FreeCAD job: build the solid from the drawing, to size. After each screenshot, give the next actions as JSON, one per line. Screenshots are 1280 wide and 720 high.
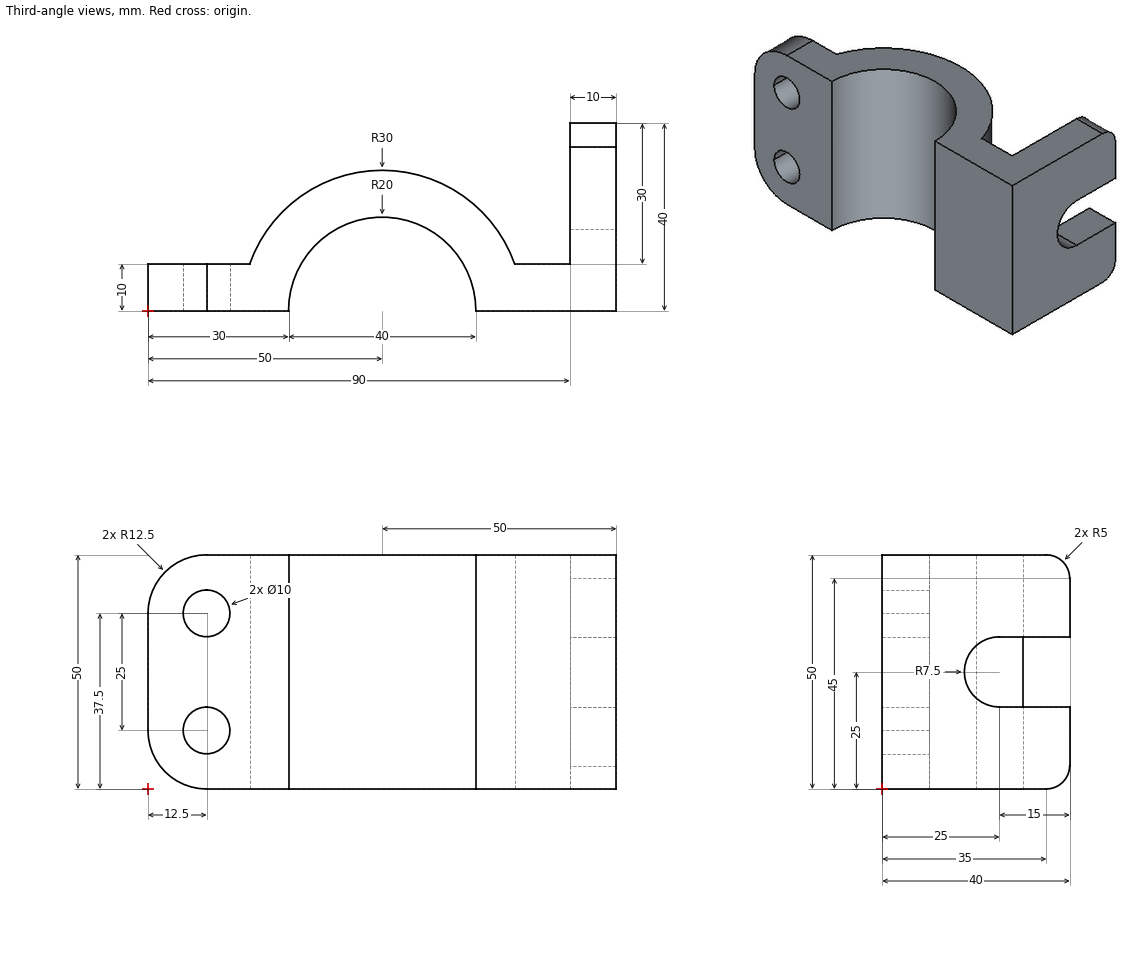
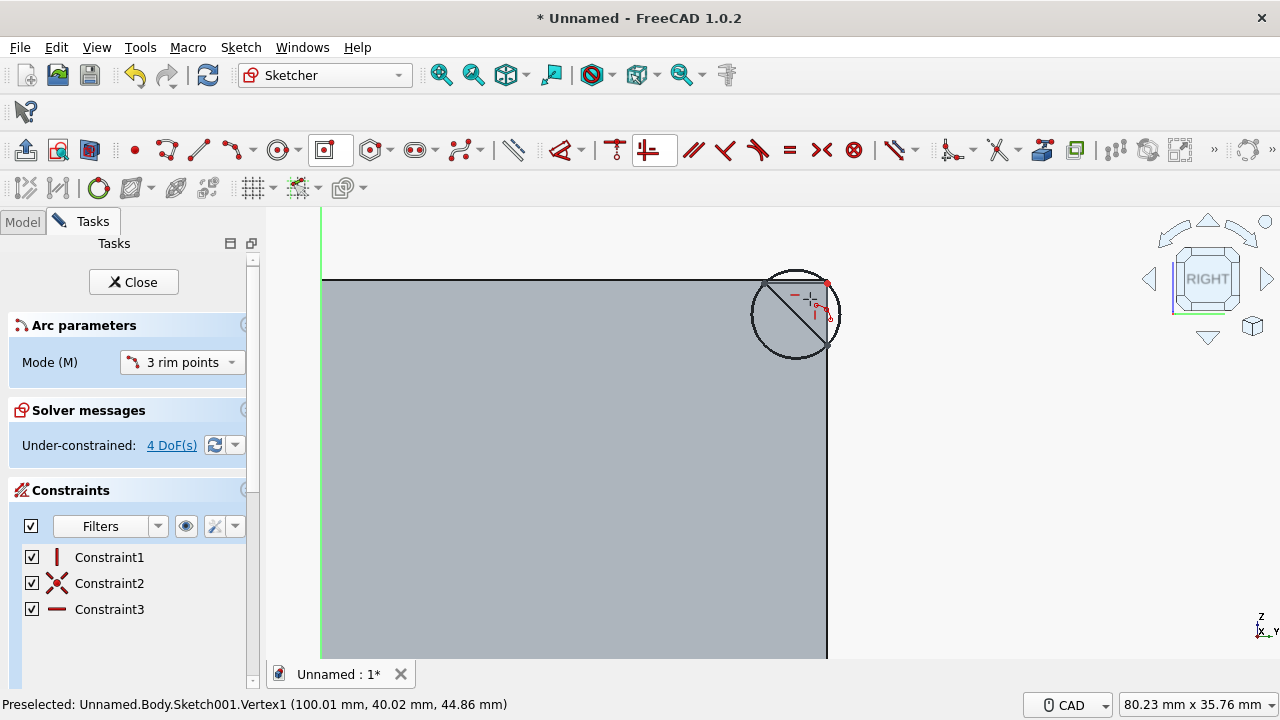
{"action": "left_click", "coordinate": [808, 299]}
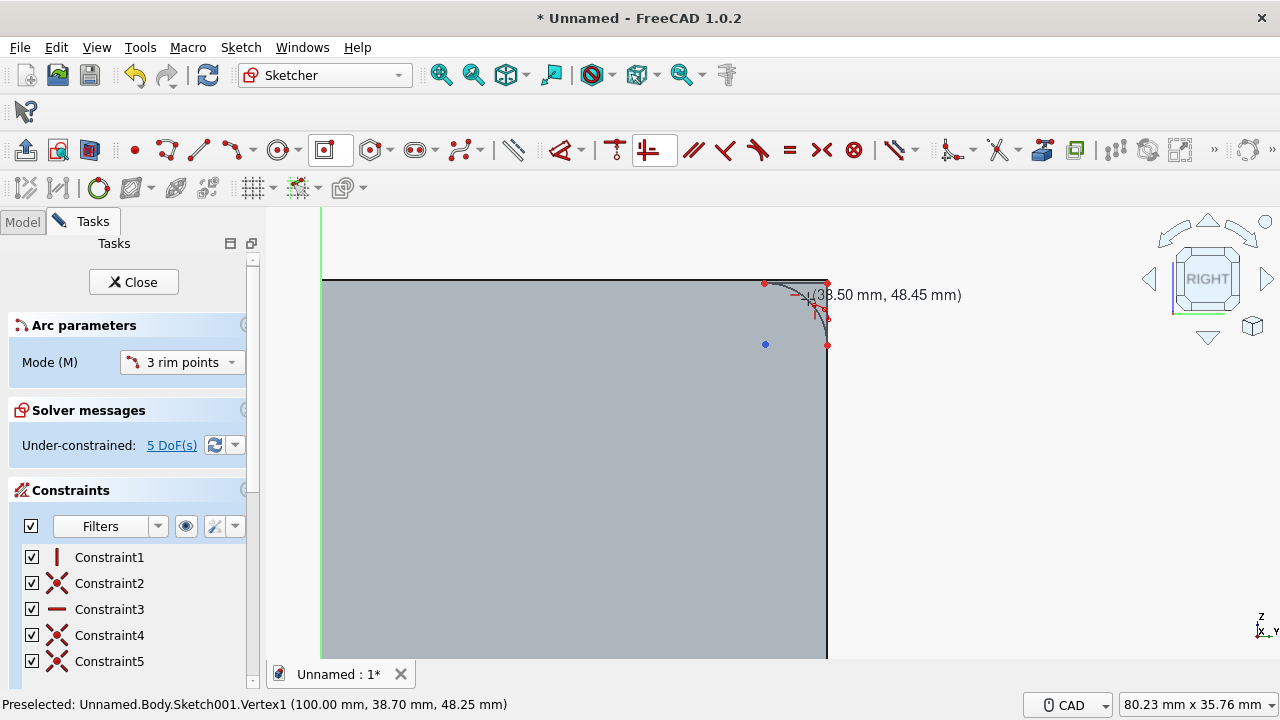
{"action": "left_click", "coordinate": [168, 150]}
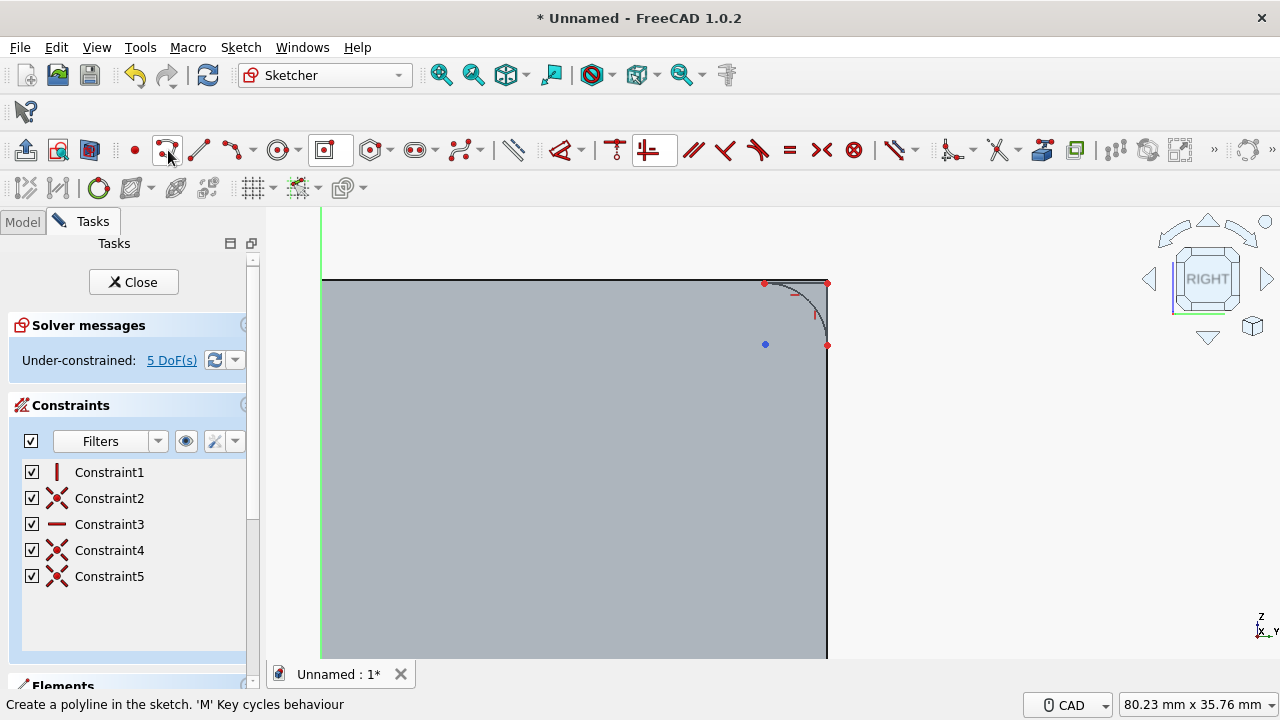
{"action": "scroll", "coordinate": [811, 300], "scroll_direction": "down", "scroll_amount": 4}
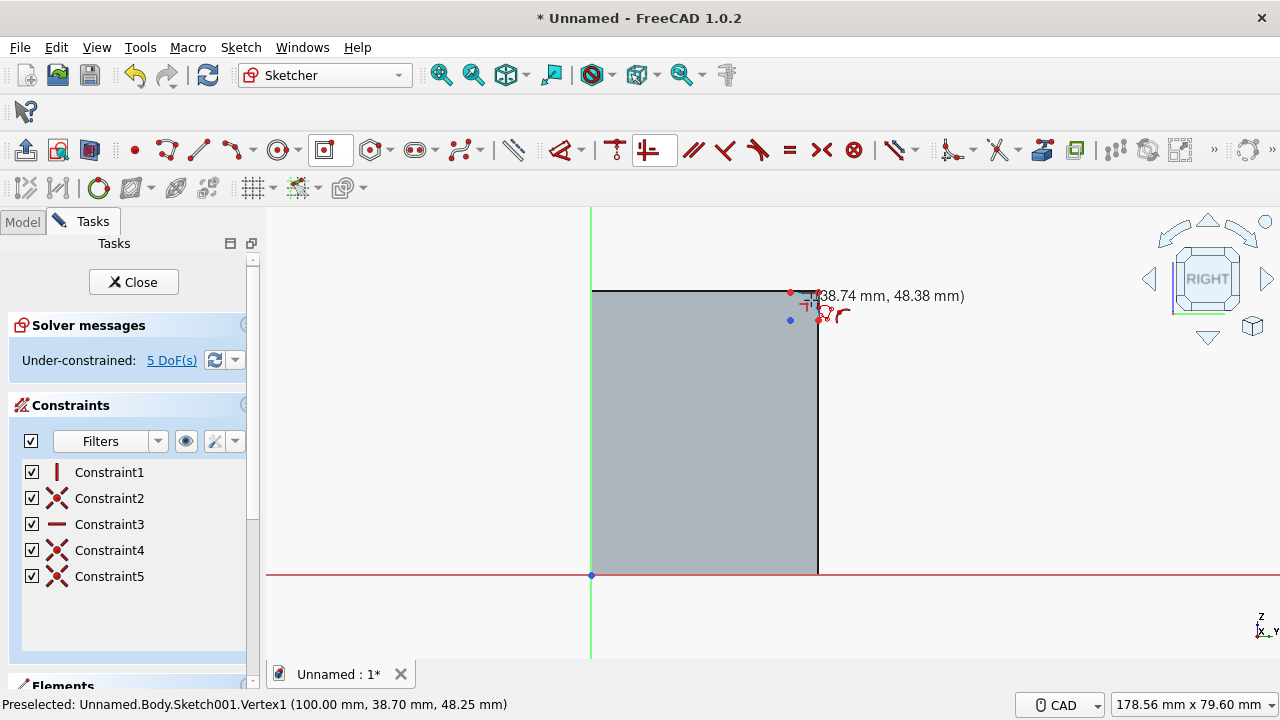
{"action": "left_click", "coordinate": [790, 575]}
{"action": "left_click", "coordinate": [818, 566]}
{"action": "left_click", "coordinate": [818, 547]}
{"action": "right_click", "coordinate": [818, 547]}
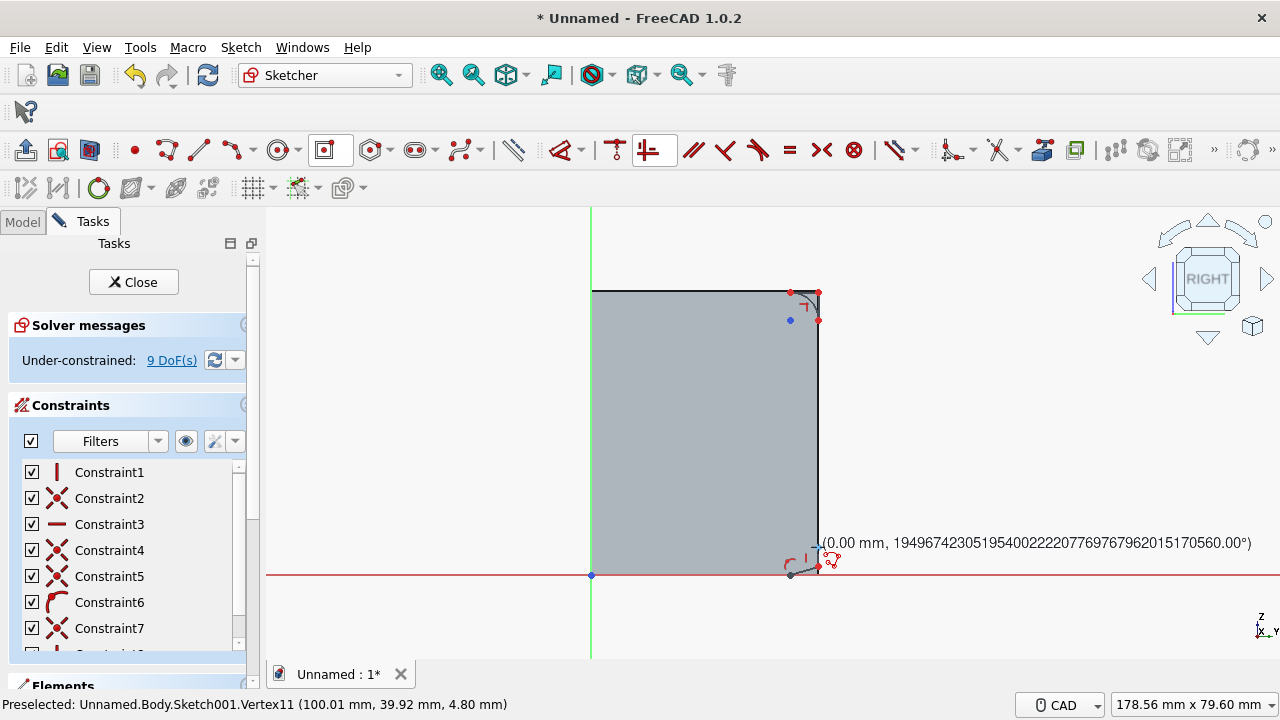
{"action": "left_click", "coordinate": [232, 150]}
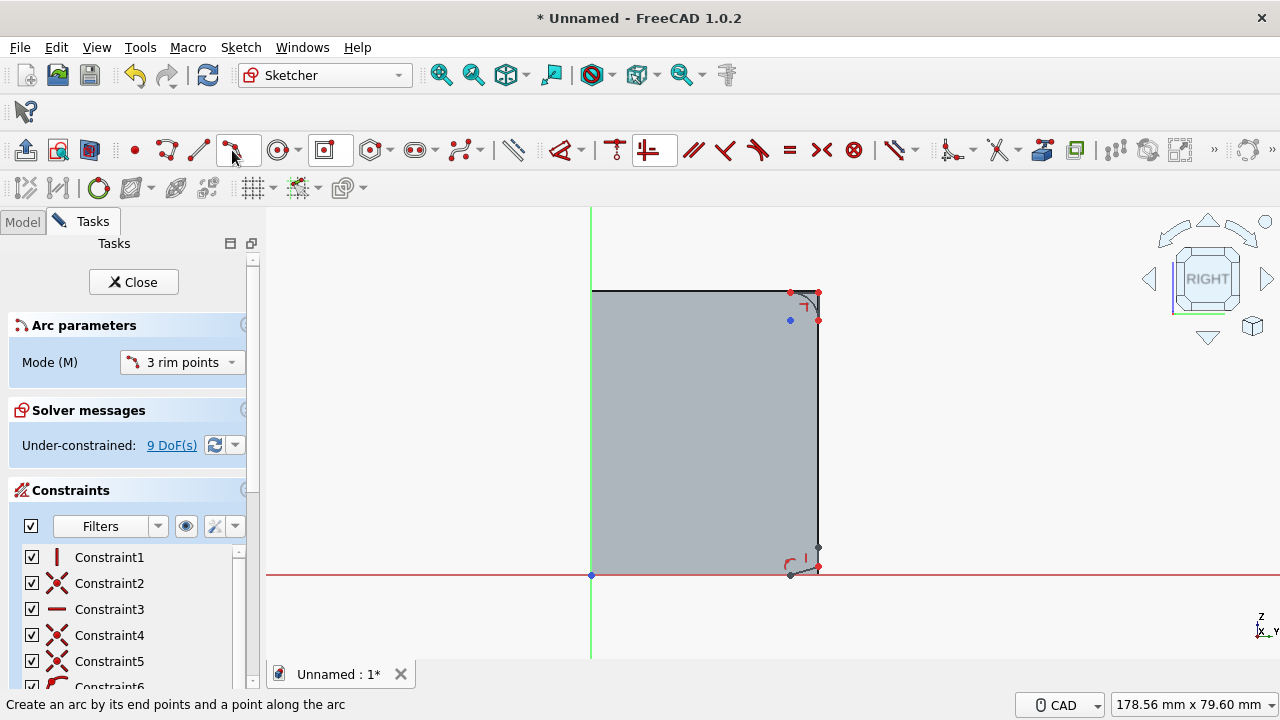
{"action": "left_click", "coordinate": [818, 548]}
{"action": "left_click", "coordinate": [790, 575]}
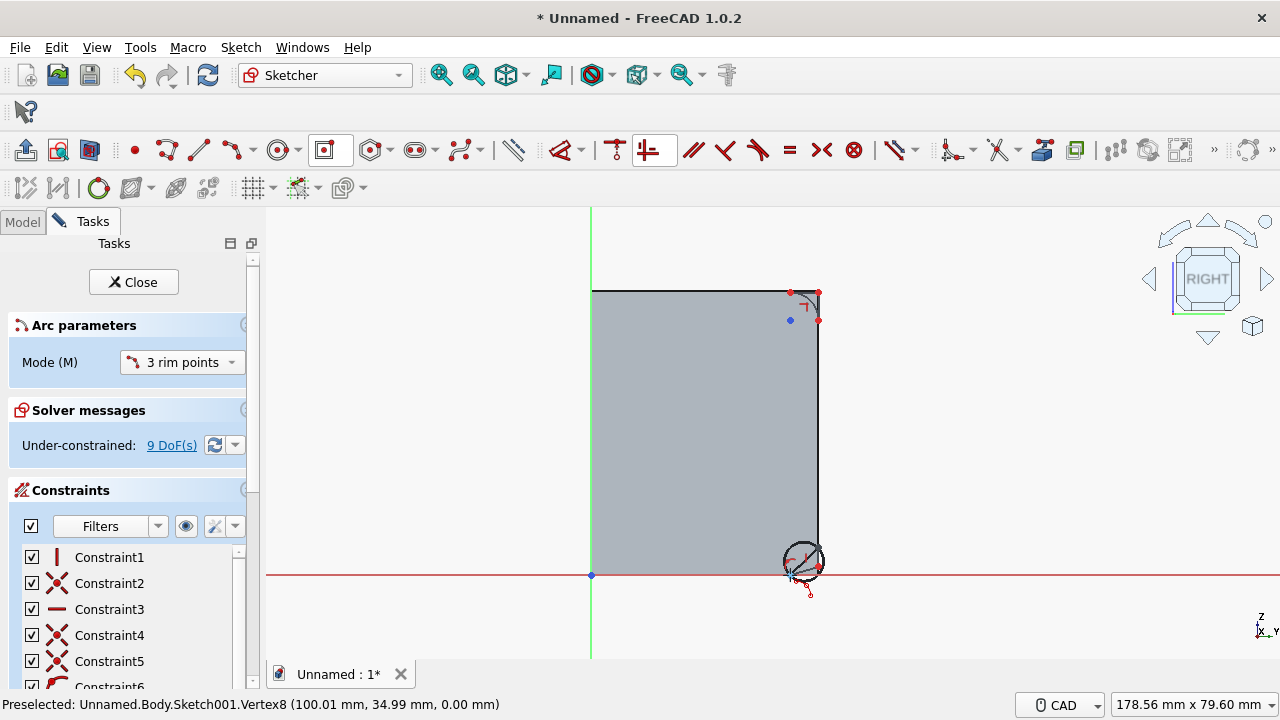
{"action": "scroll", "coordinate": [810, 567], "scroll_direction": "up", "scroll_amount": 4}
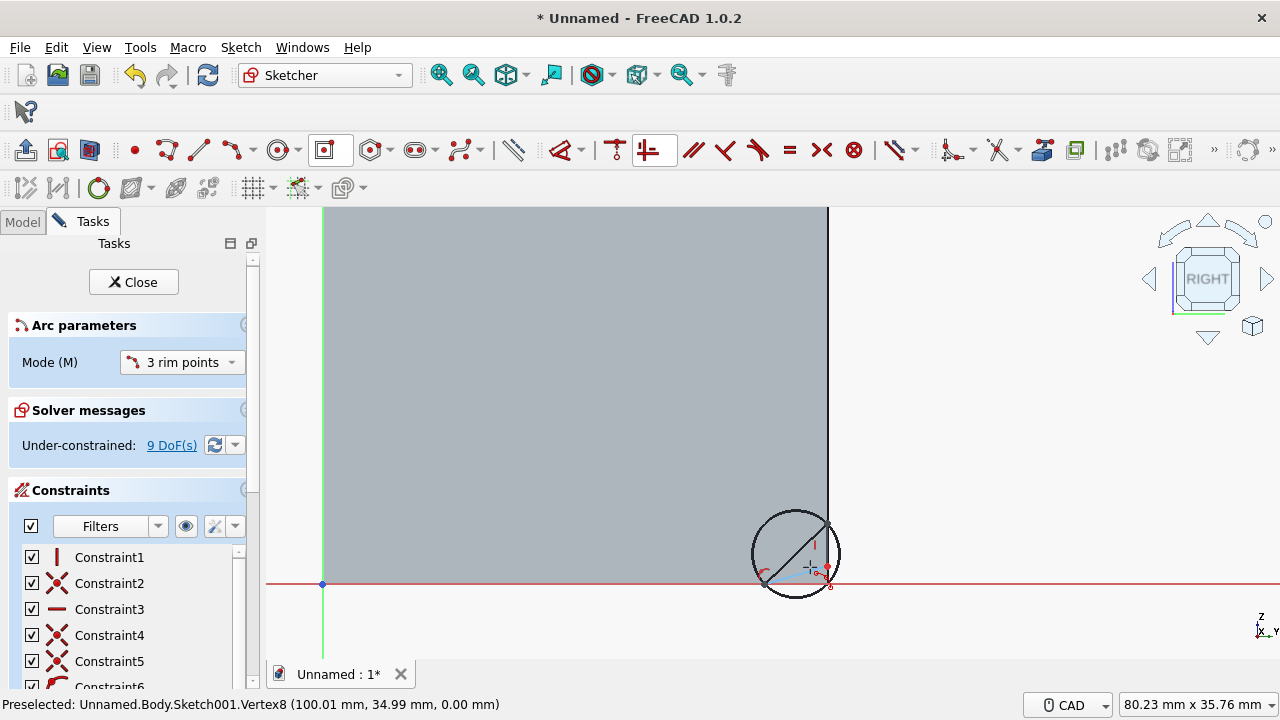
{"action": "left_click", "coordinate": [810, 566]}
{"action": "key", "text": "Escape"}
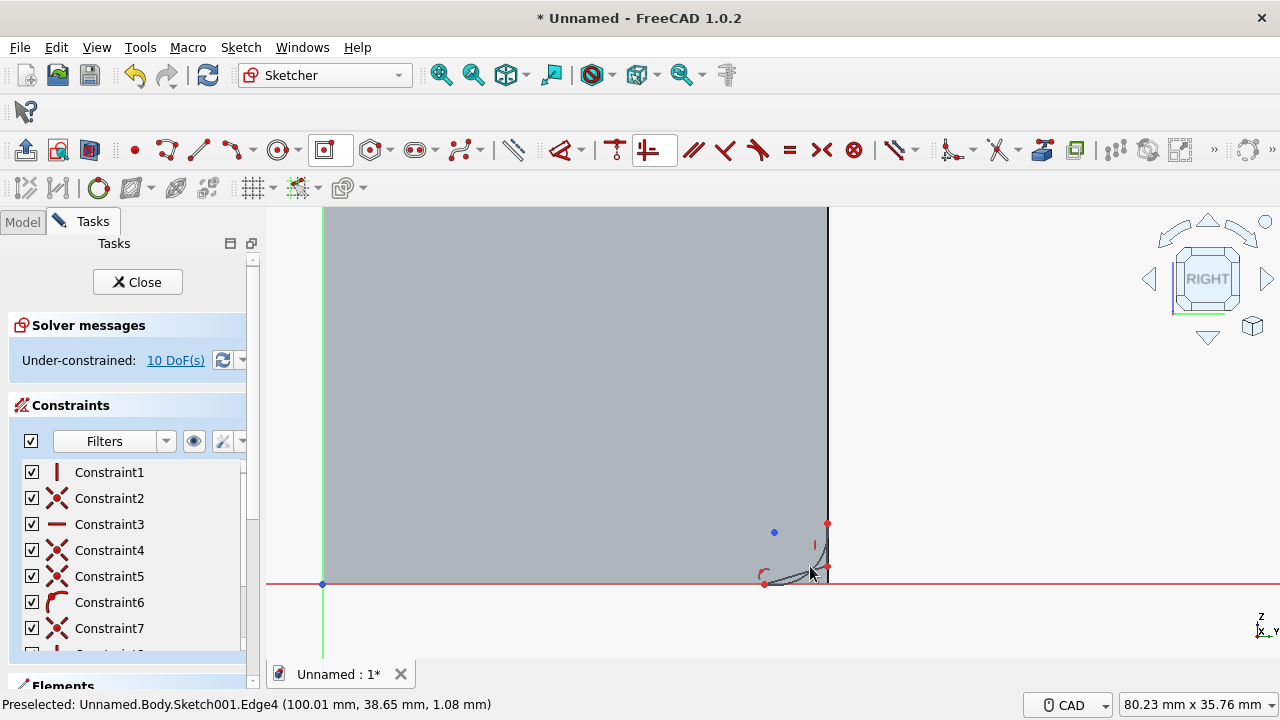
{"action": "scroll", "coordinate": [810, 567], "scroll_direction": "down", "scroll_amount": 4}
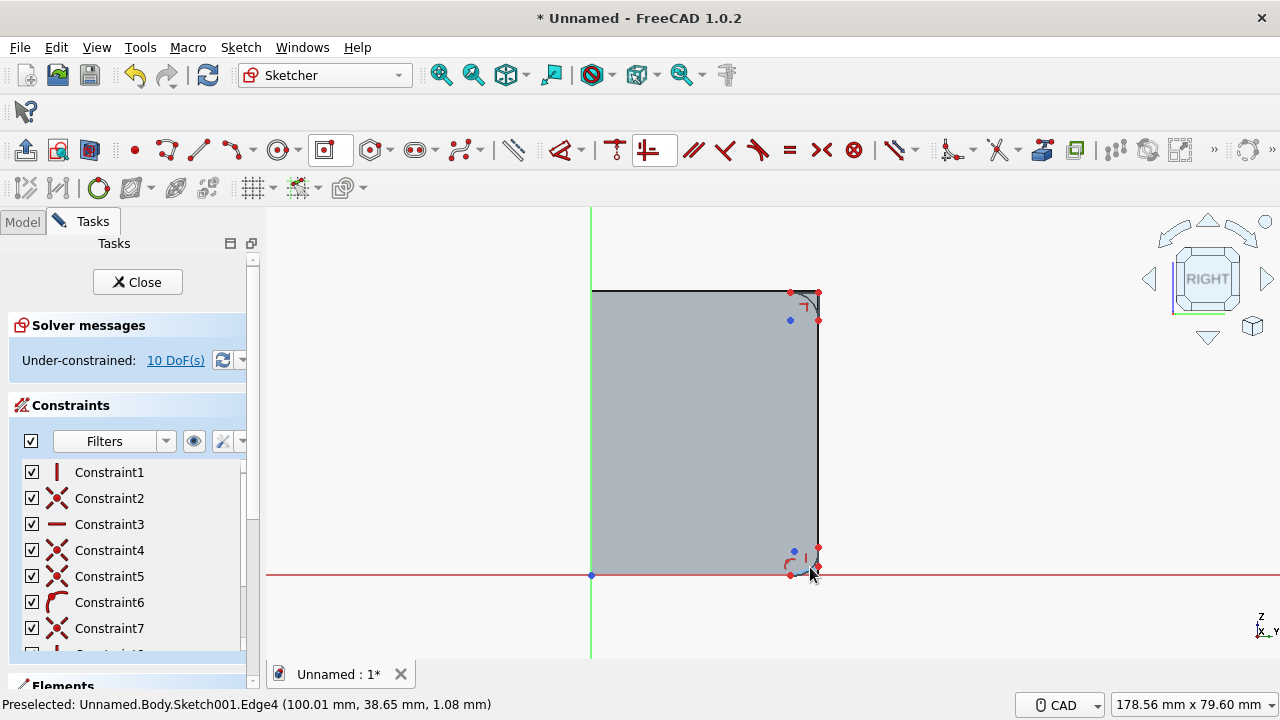
{"action": "scroll", "coordinate": [819, 301], "scroll_direction": "up", "scroll_amount": 5}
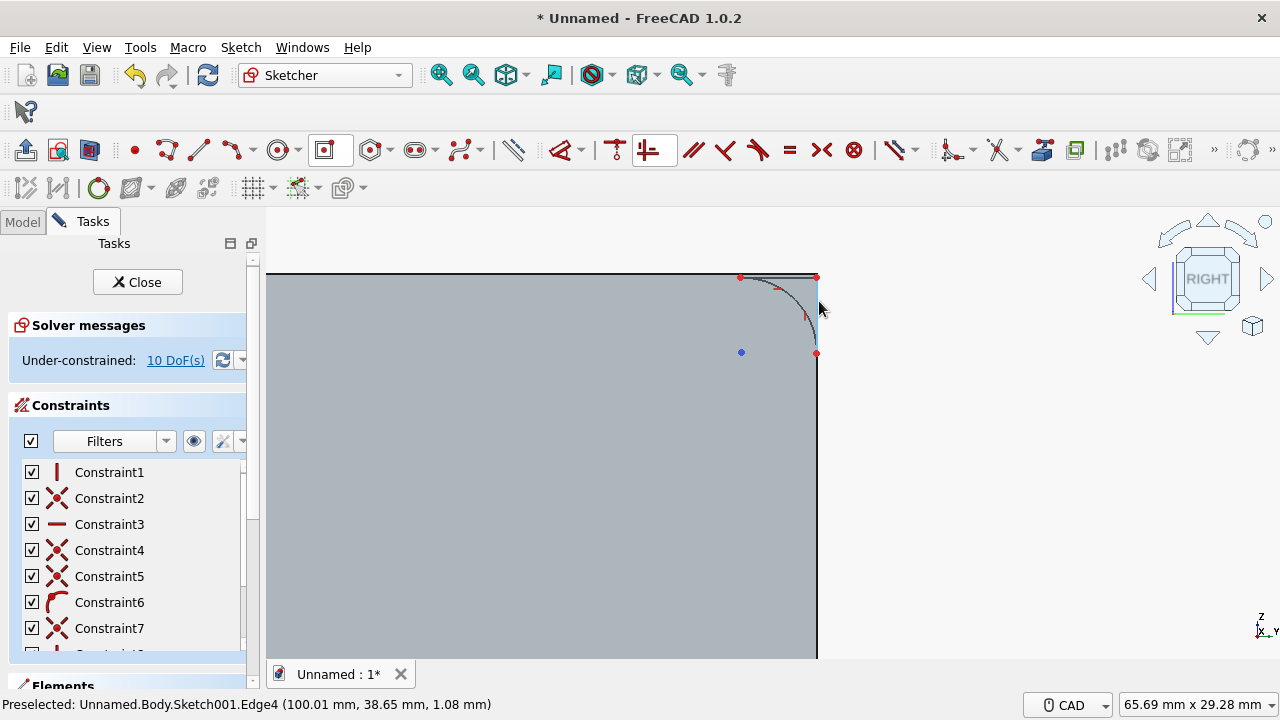
{"action": "left_click", "coordinate": [817, 301]}